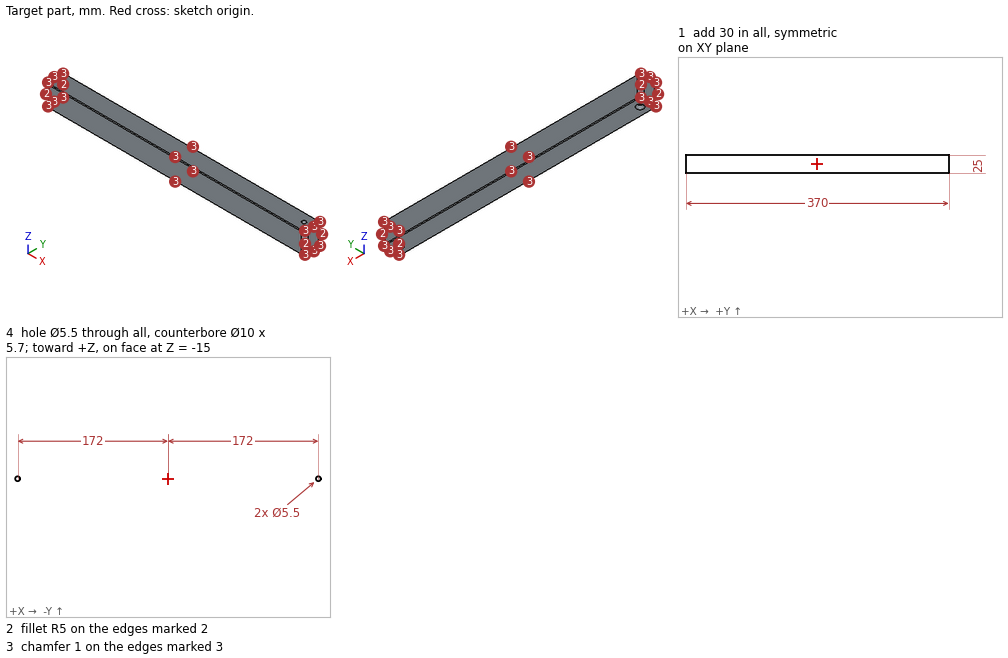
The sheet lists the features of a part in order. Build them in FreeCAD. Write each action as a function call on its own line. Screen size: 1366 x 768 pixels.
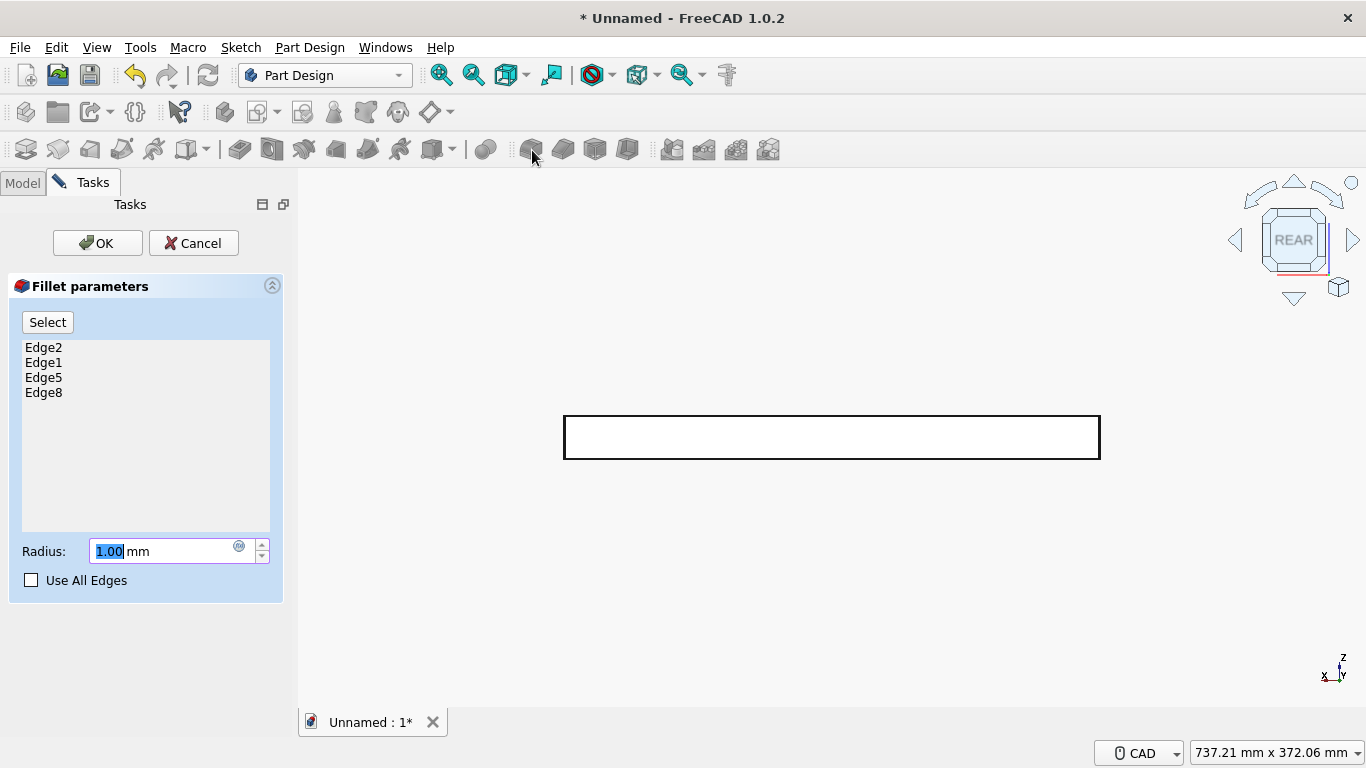
text(5)
key(Tab)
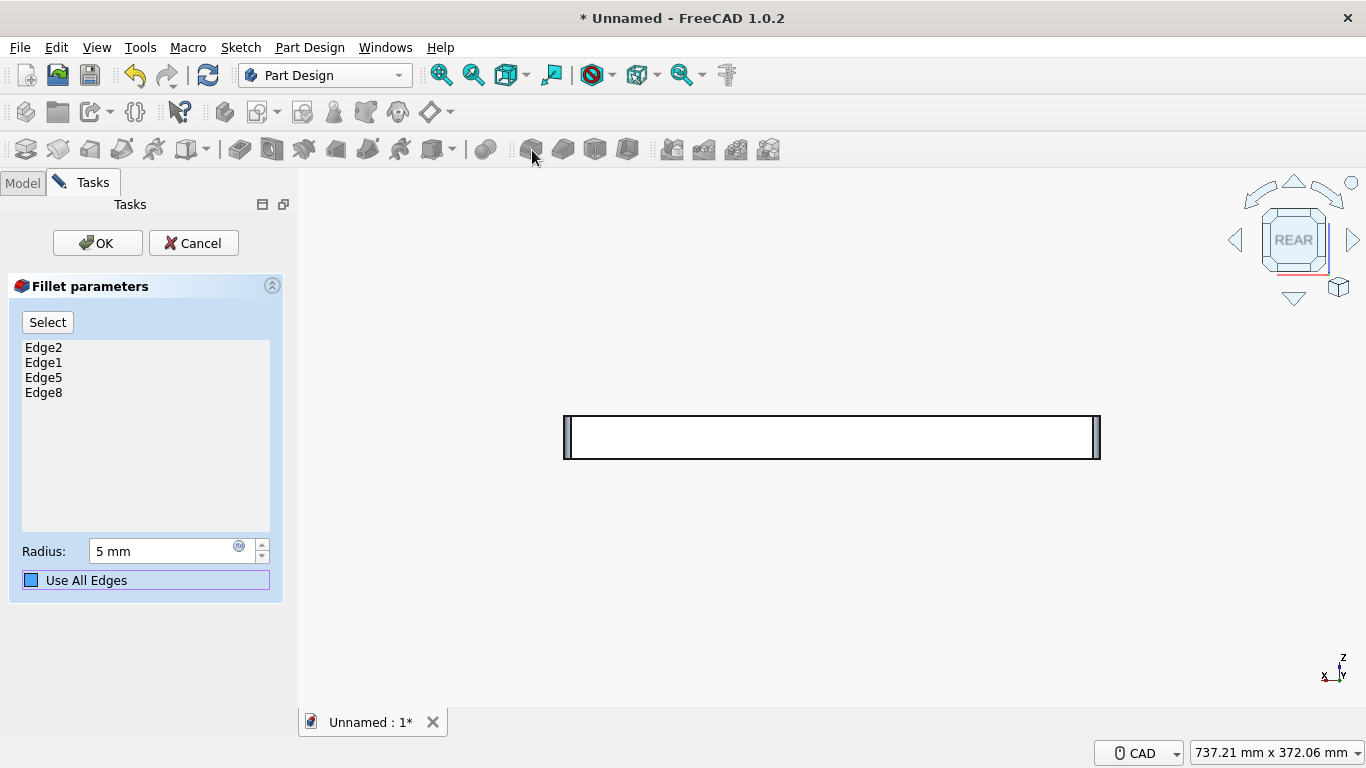
click(98, 243)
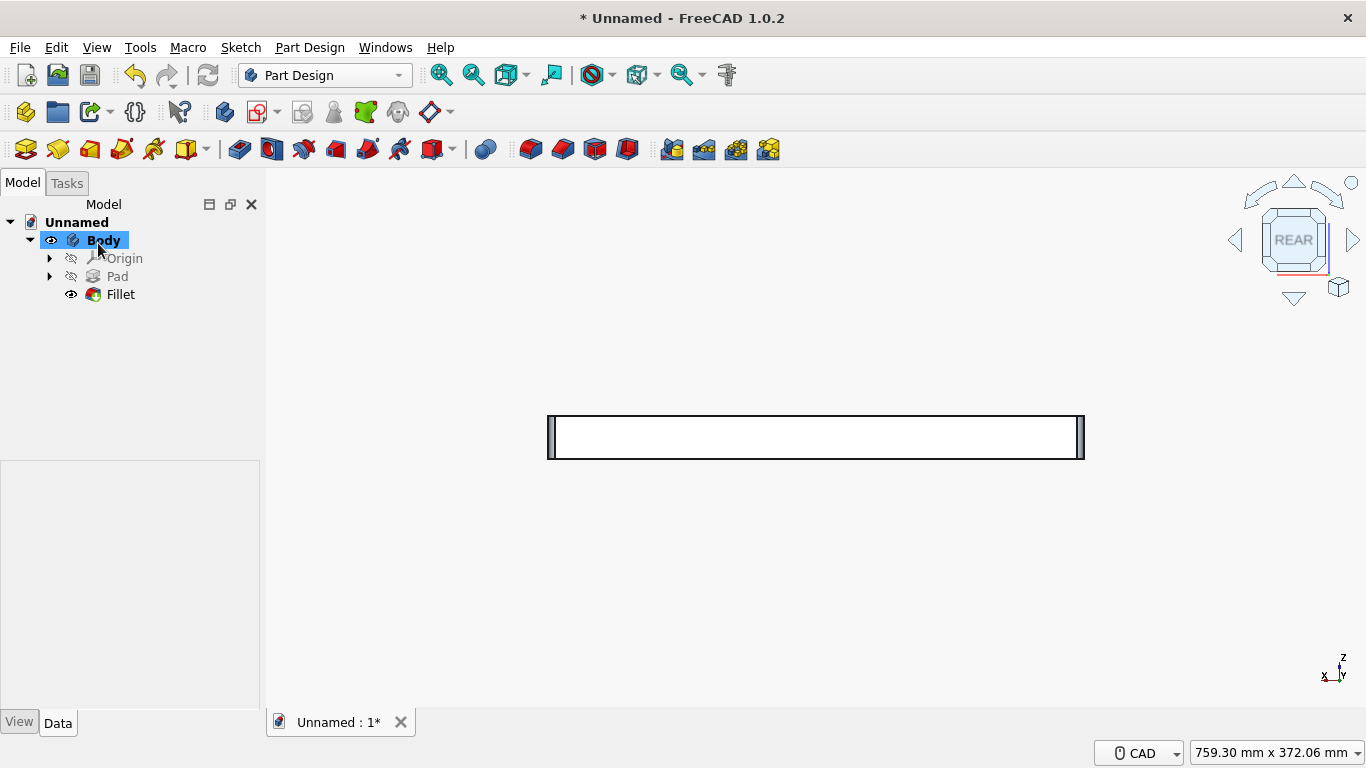
key(0)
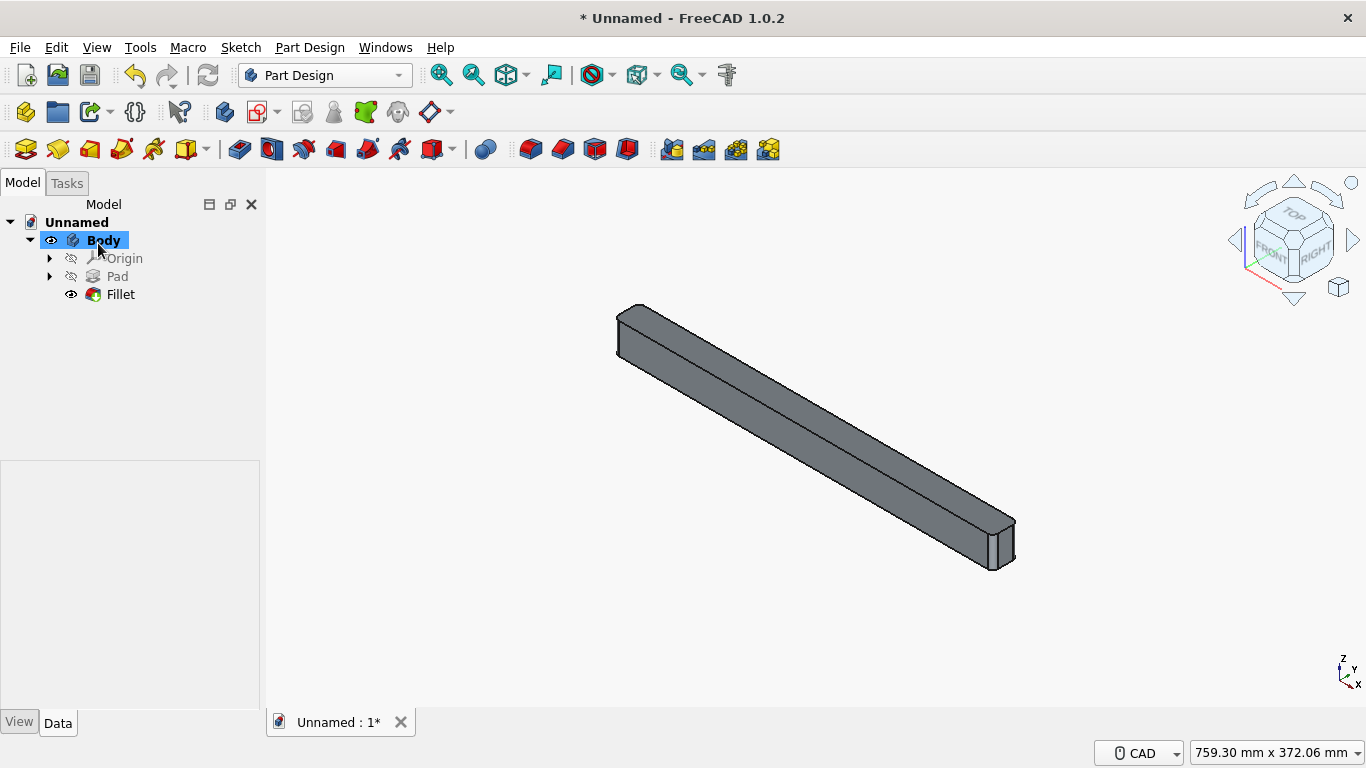
click(978, 513)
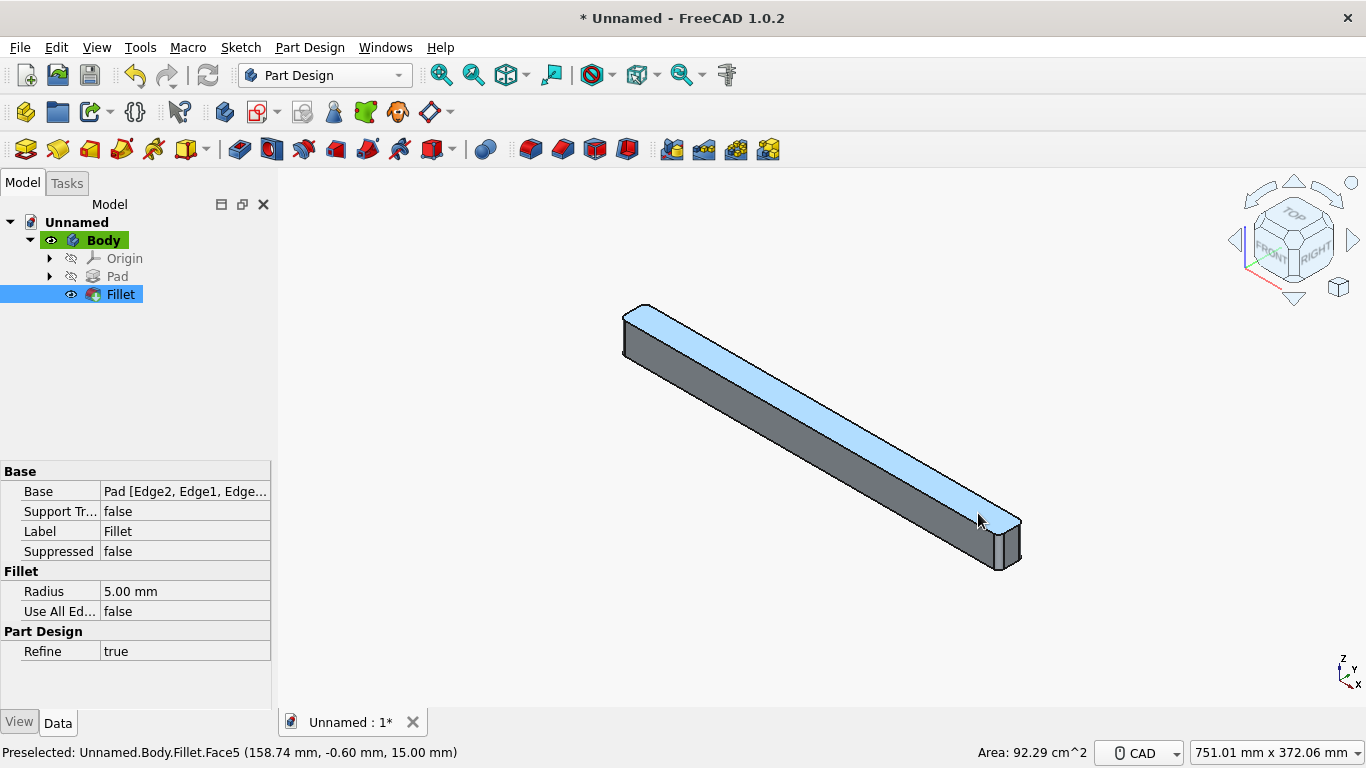
key(2)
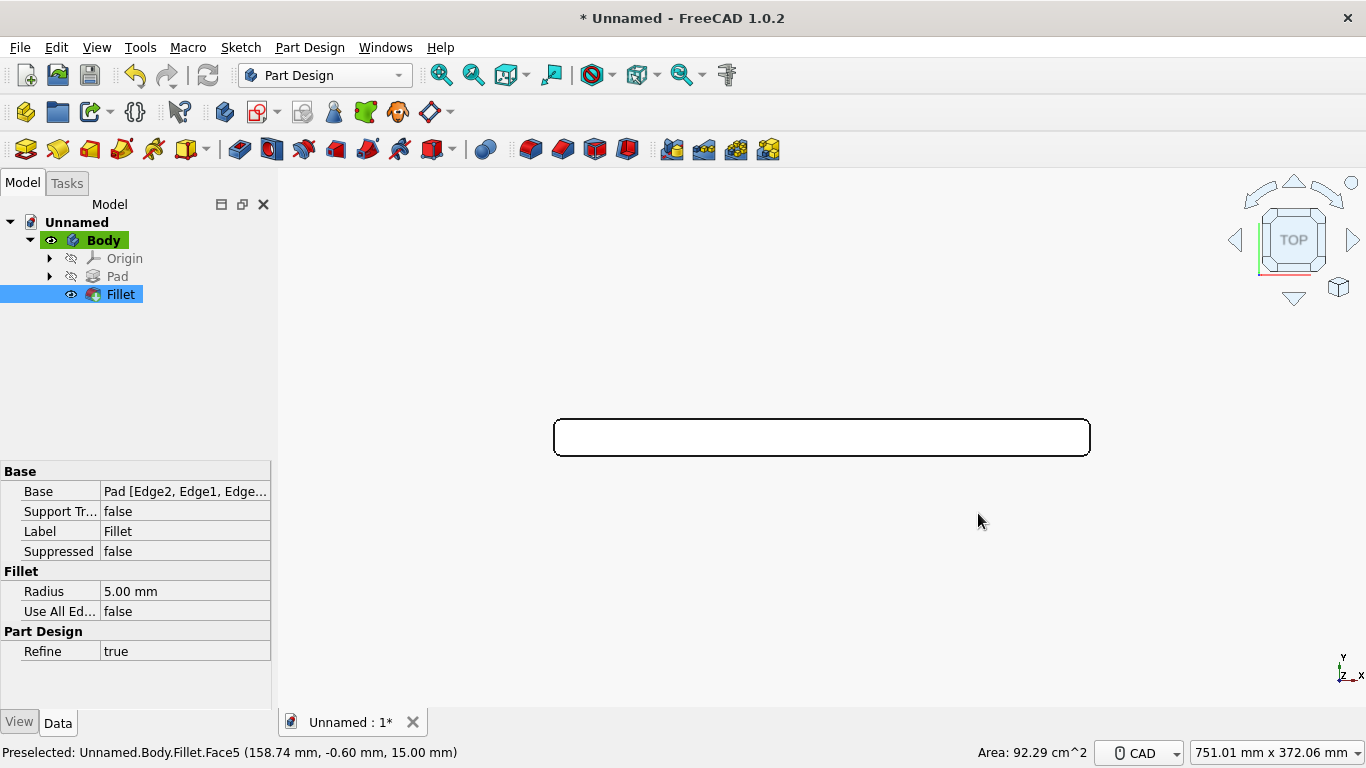
key(1)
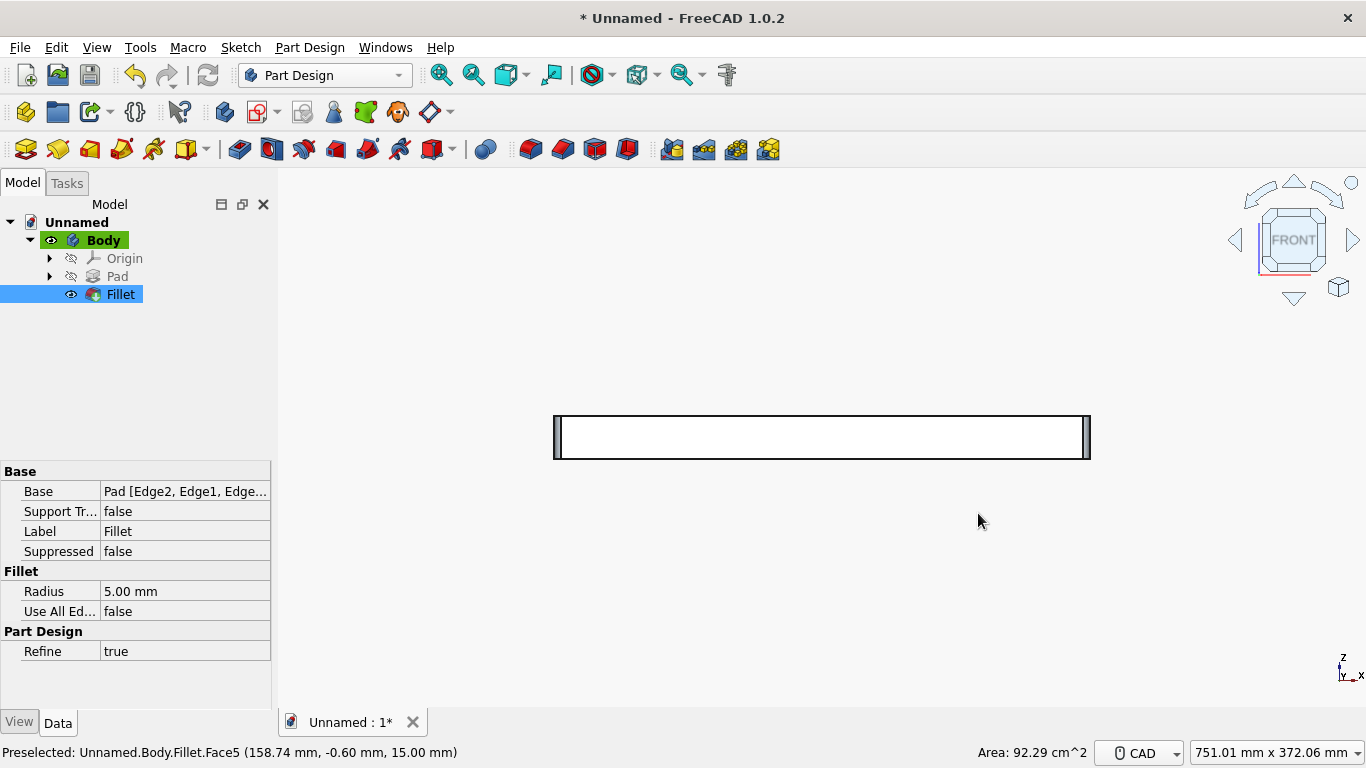
key(3)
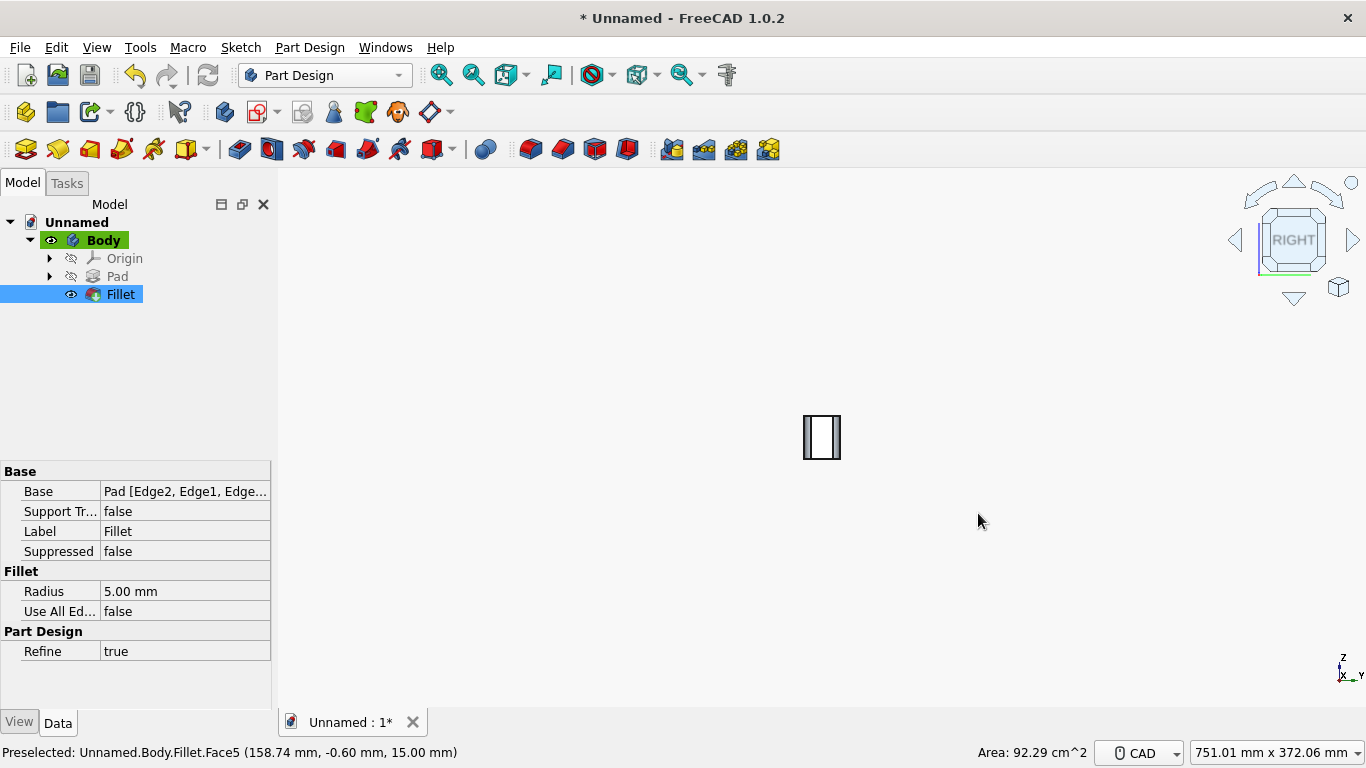
click(442, 76)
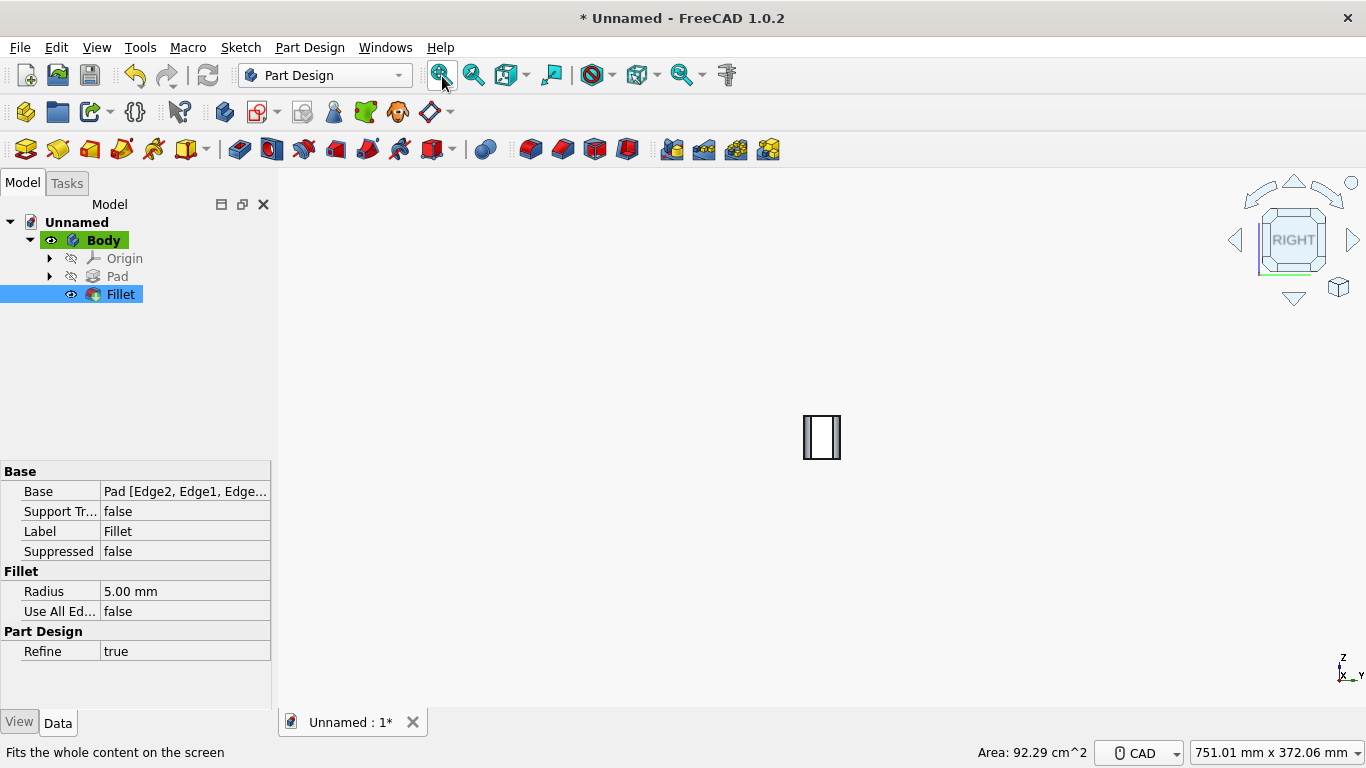
key(5)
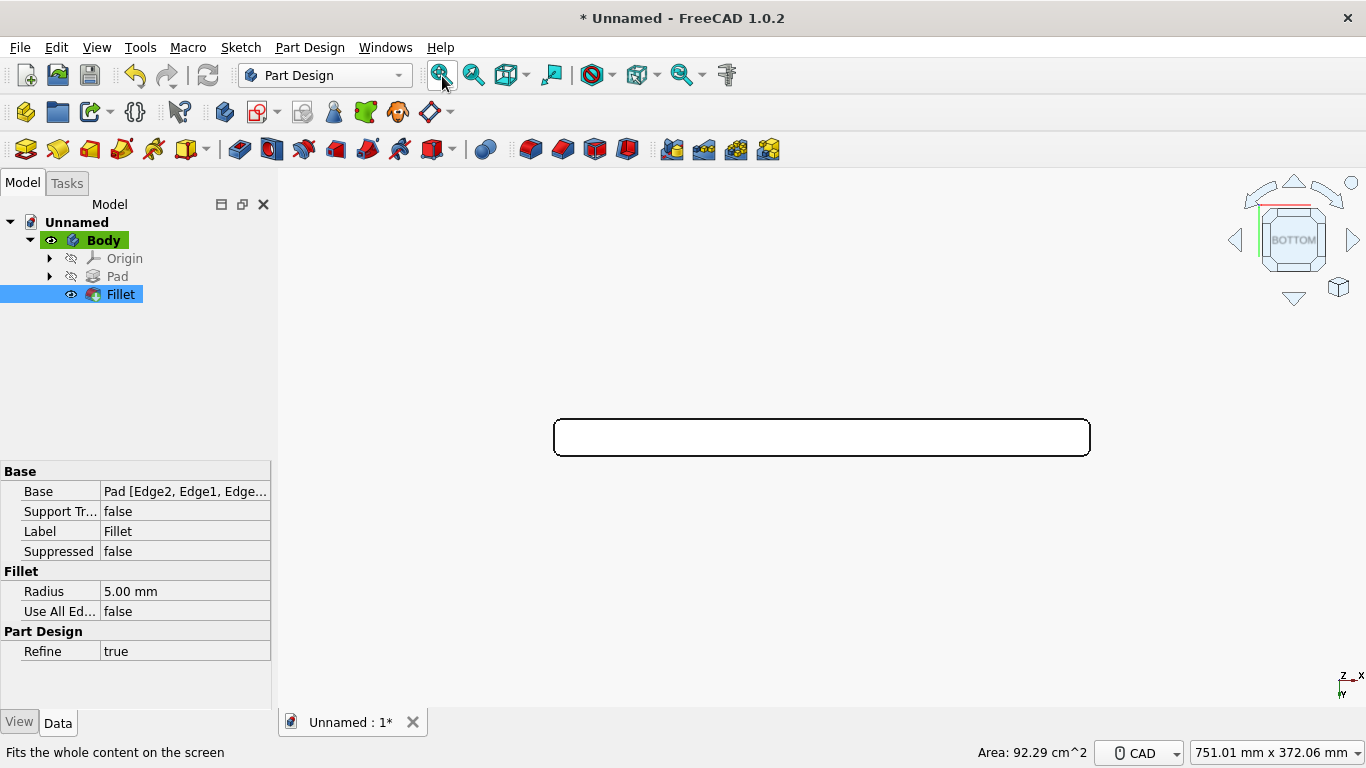
click(1052, 436, ctrl)